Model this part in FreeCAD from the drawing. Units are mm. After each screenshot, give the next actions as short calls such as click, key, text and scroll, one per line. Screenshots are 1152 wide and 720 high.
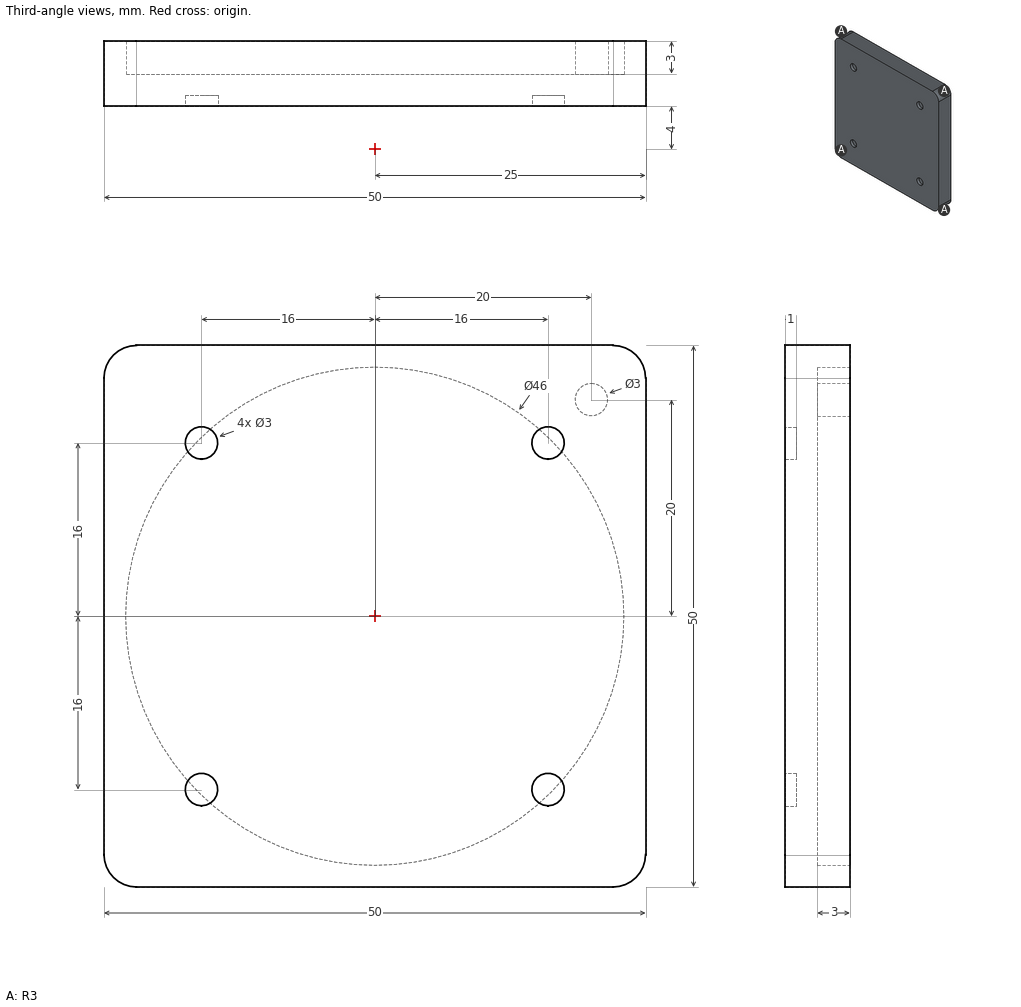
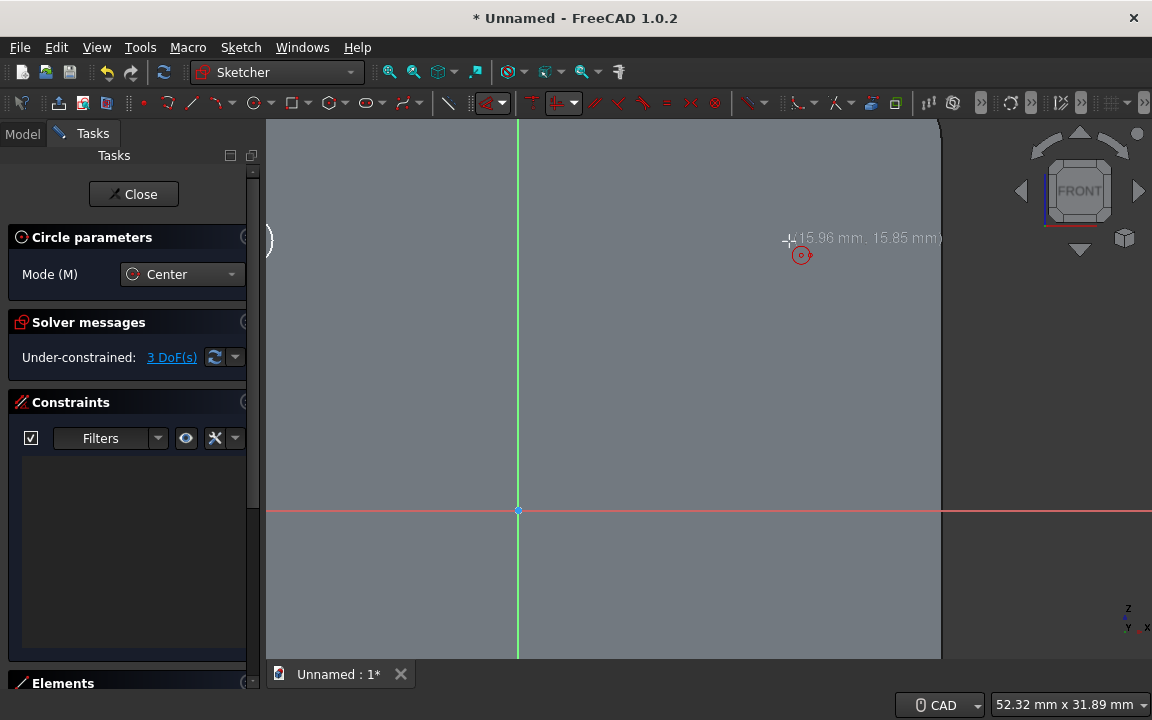
click(789, 240)
click(807, 222)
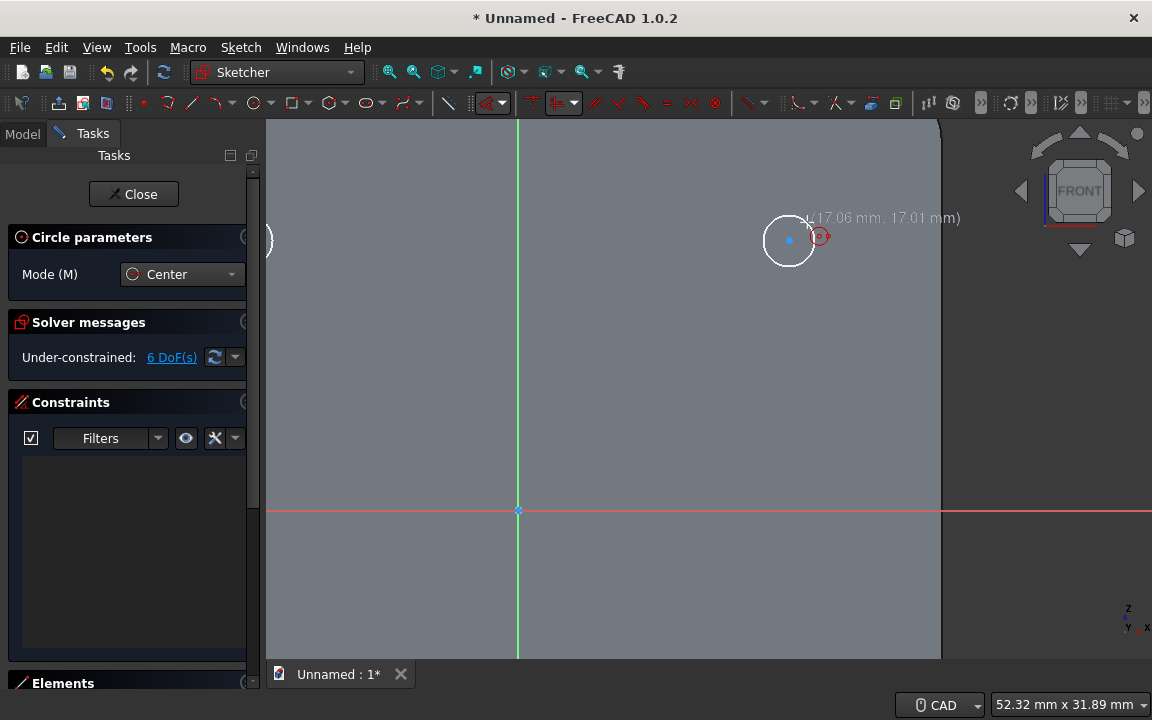
scroll(789, 241, down, 3)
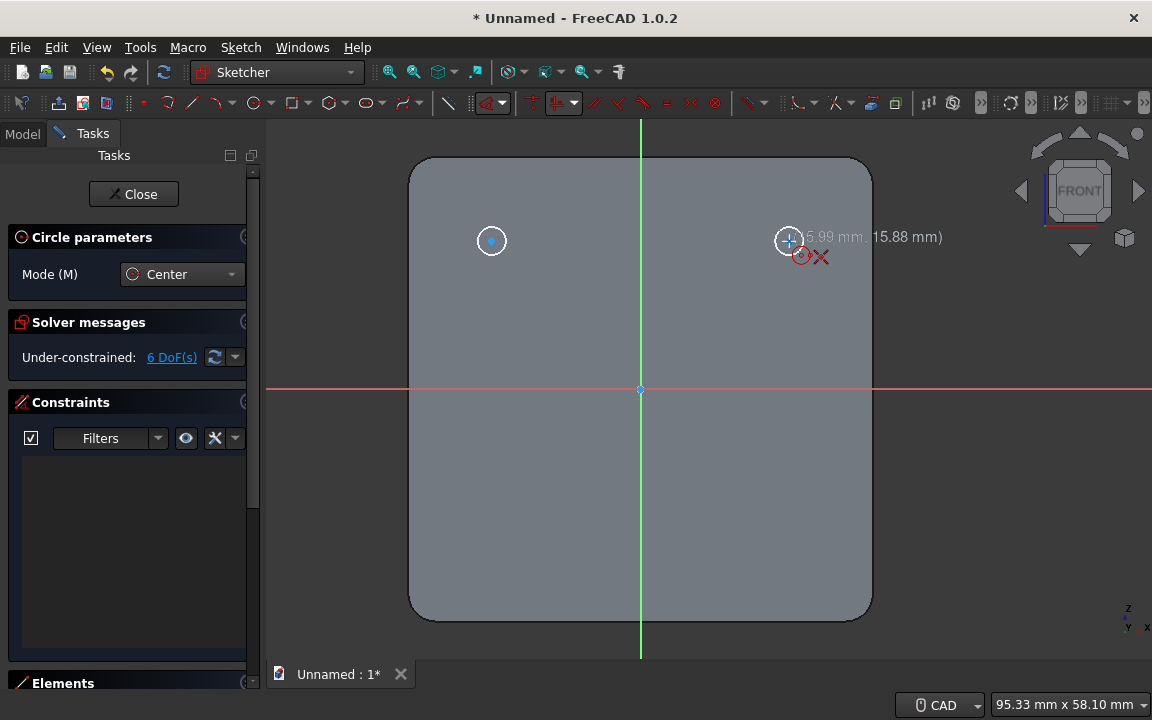
scroll(492, 538, up, 3)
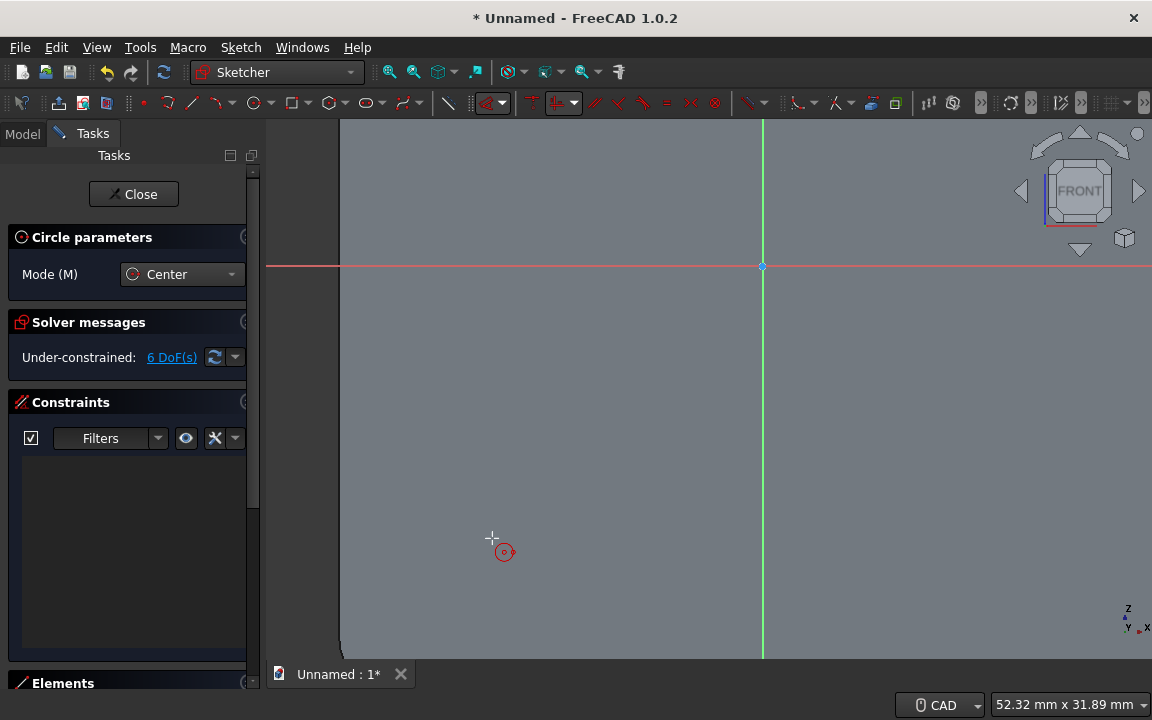
click(492, 537)
click(510, 519)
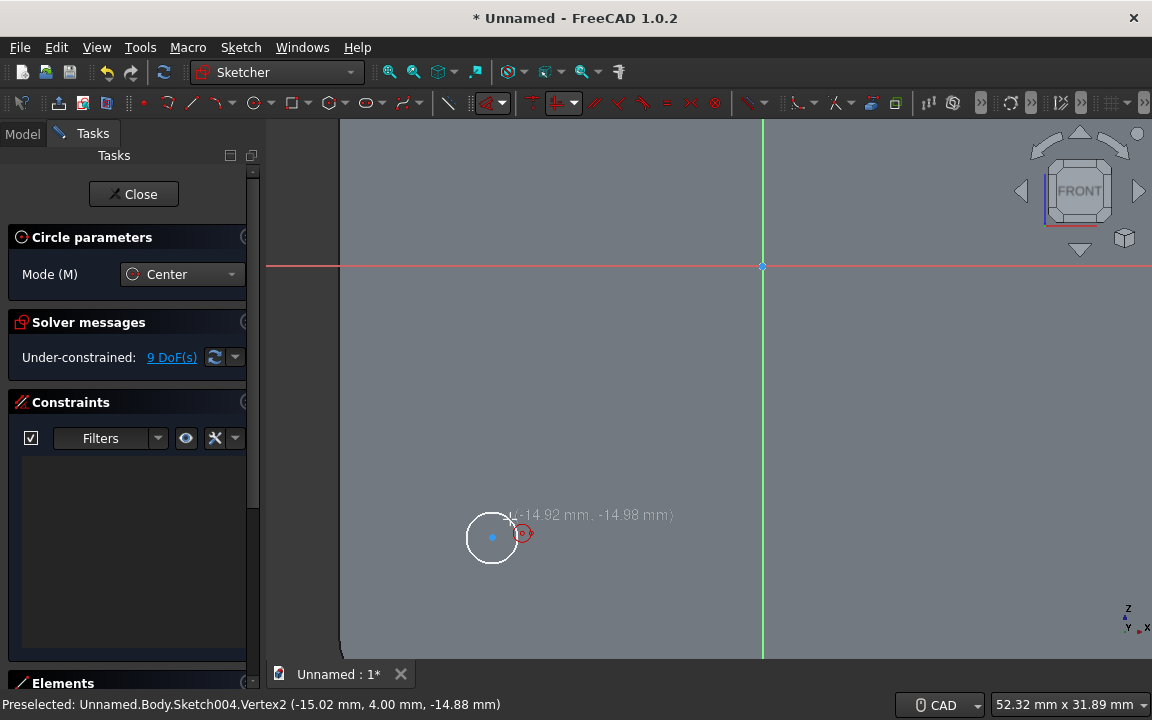
scroll(492, 538, down, 3)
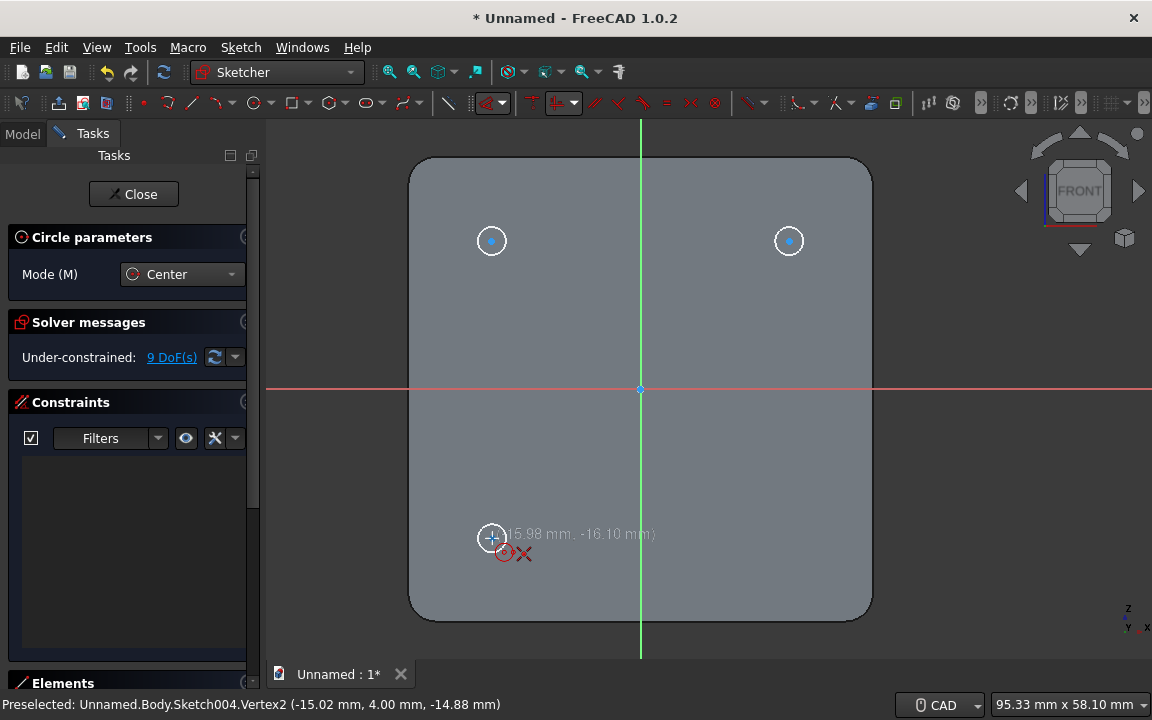
scroll(789, 538, up, 3)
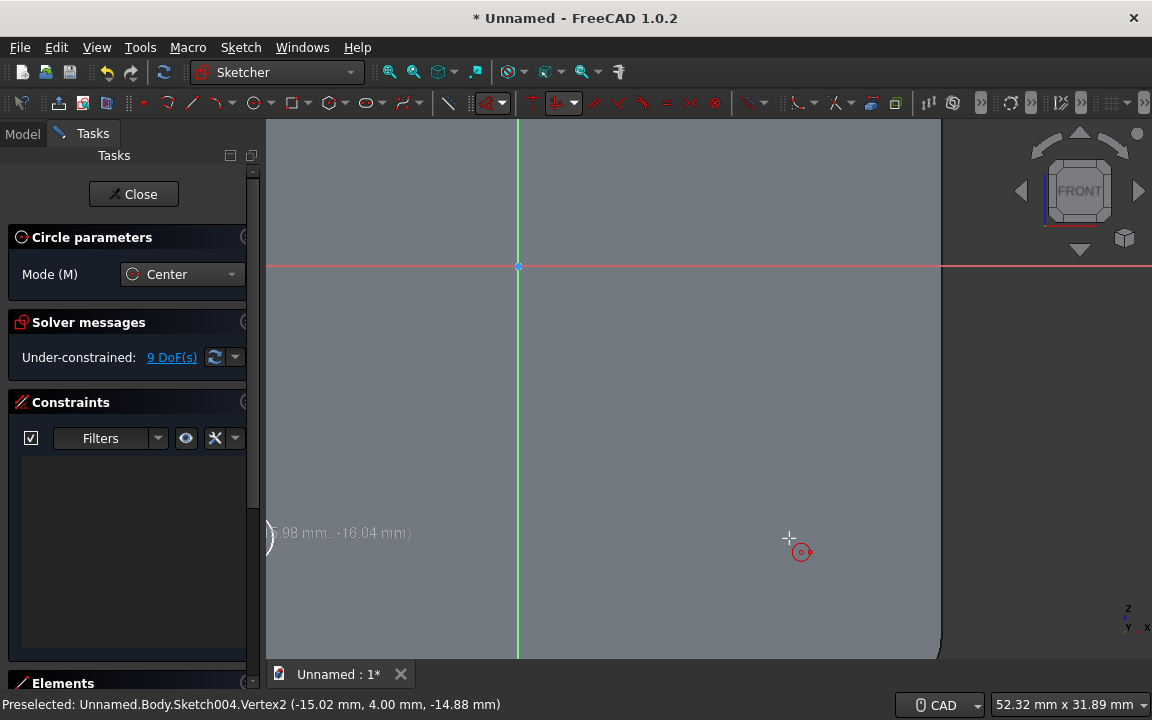
click(789, 537)
click(807, 519)
key(Escape)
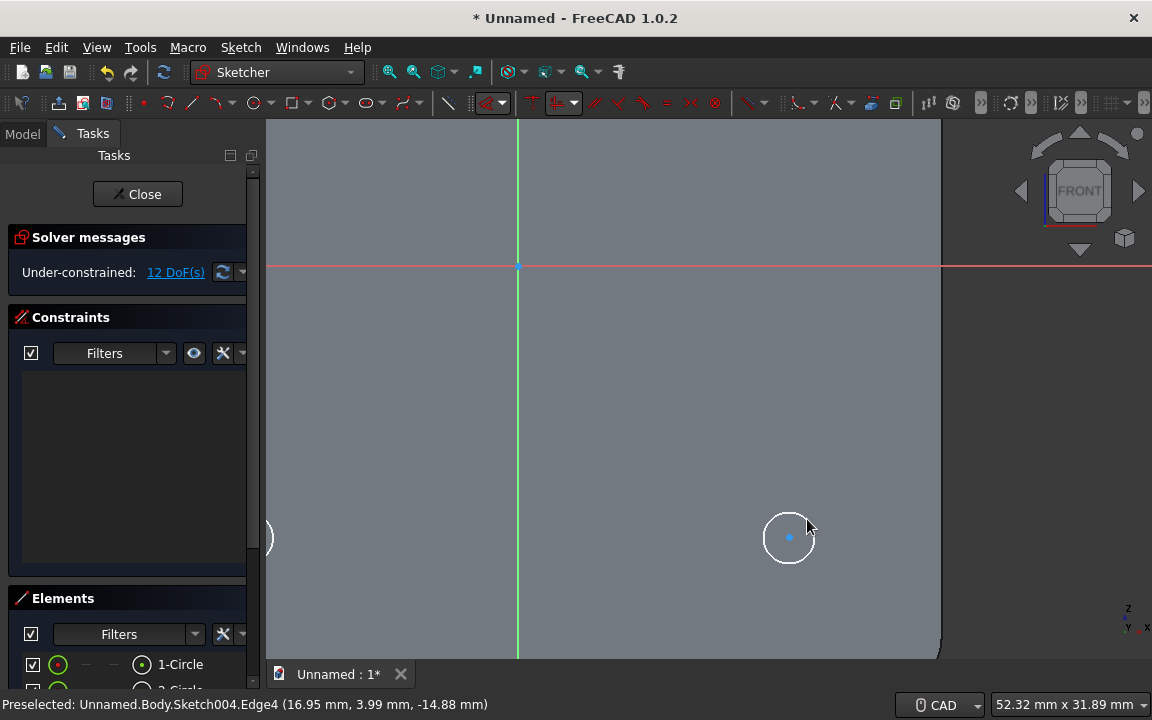
scroll(789, 538, down, 3)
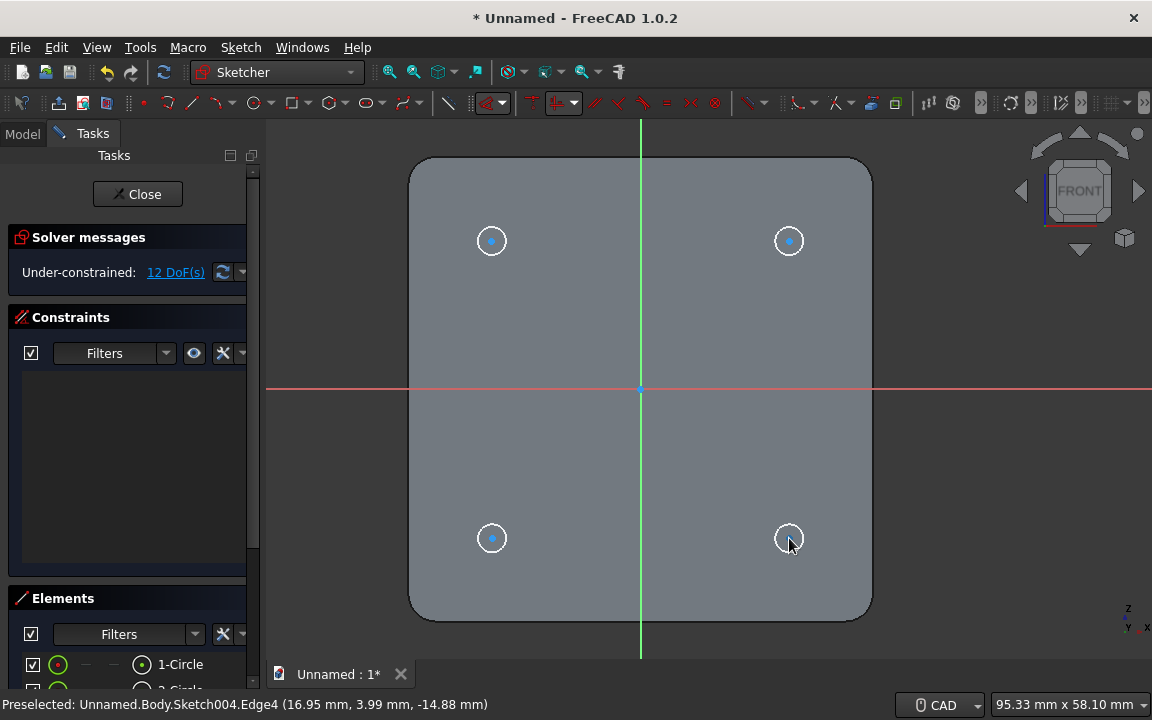
click(502, 231)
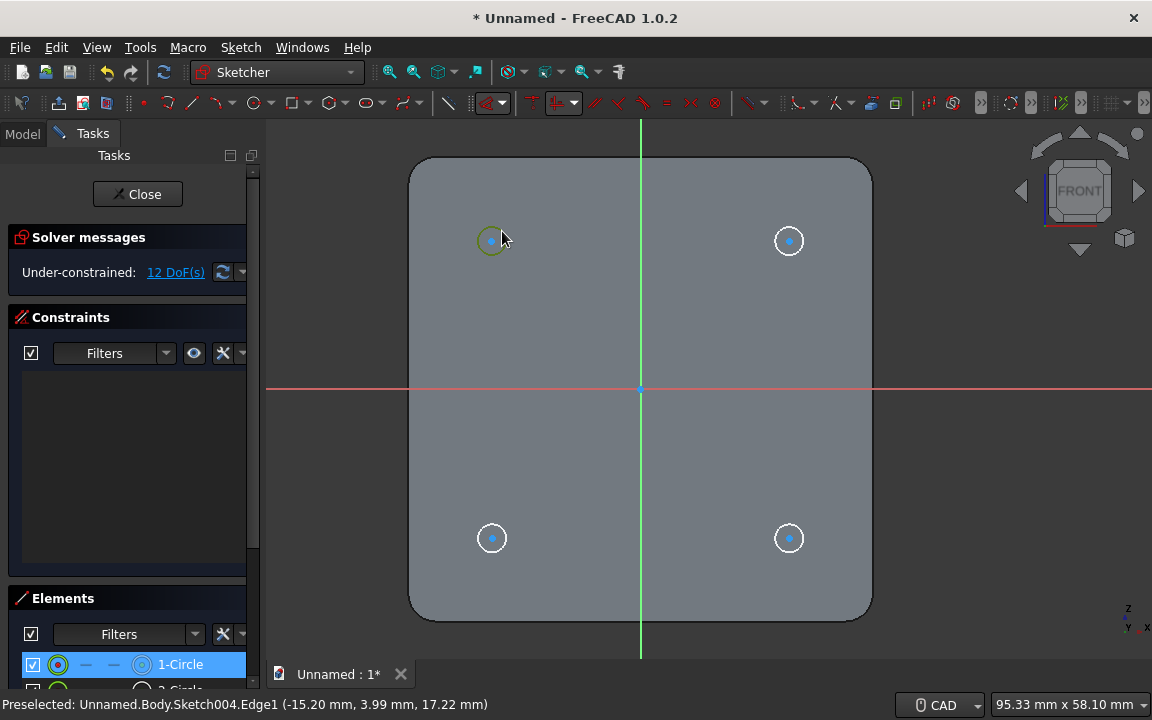
click(799, 231)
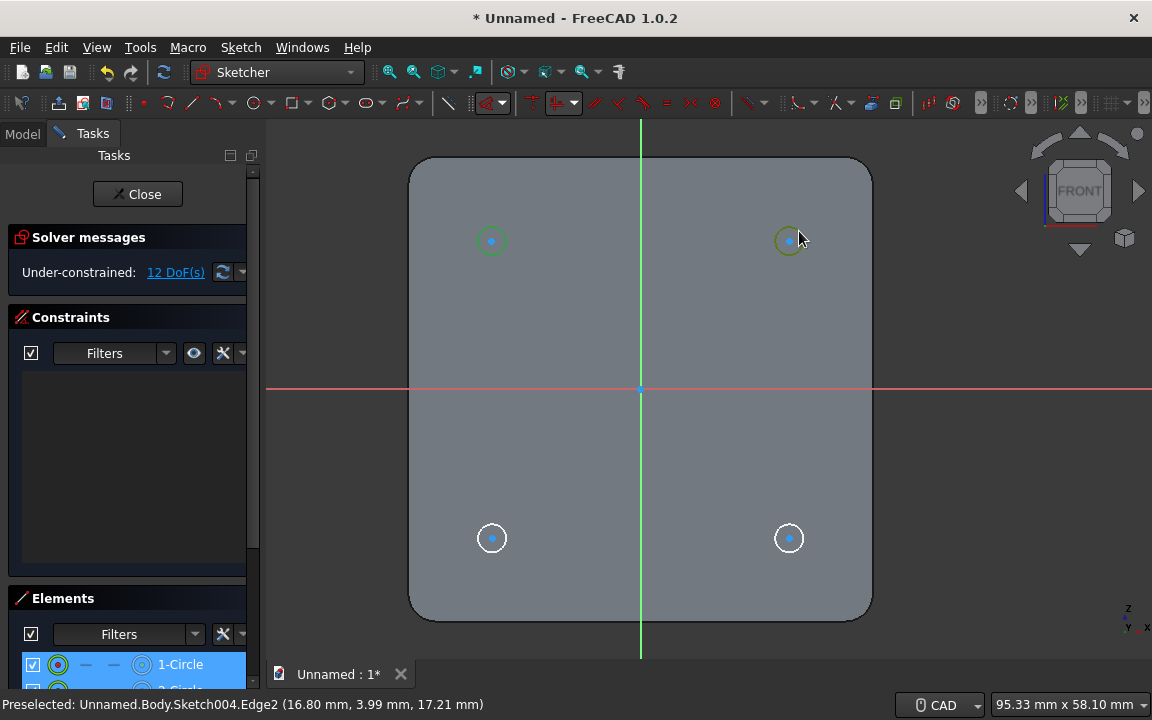
click(502, 528)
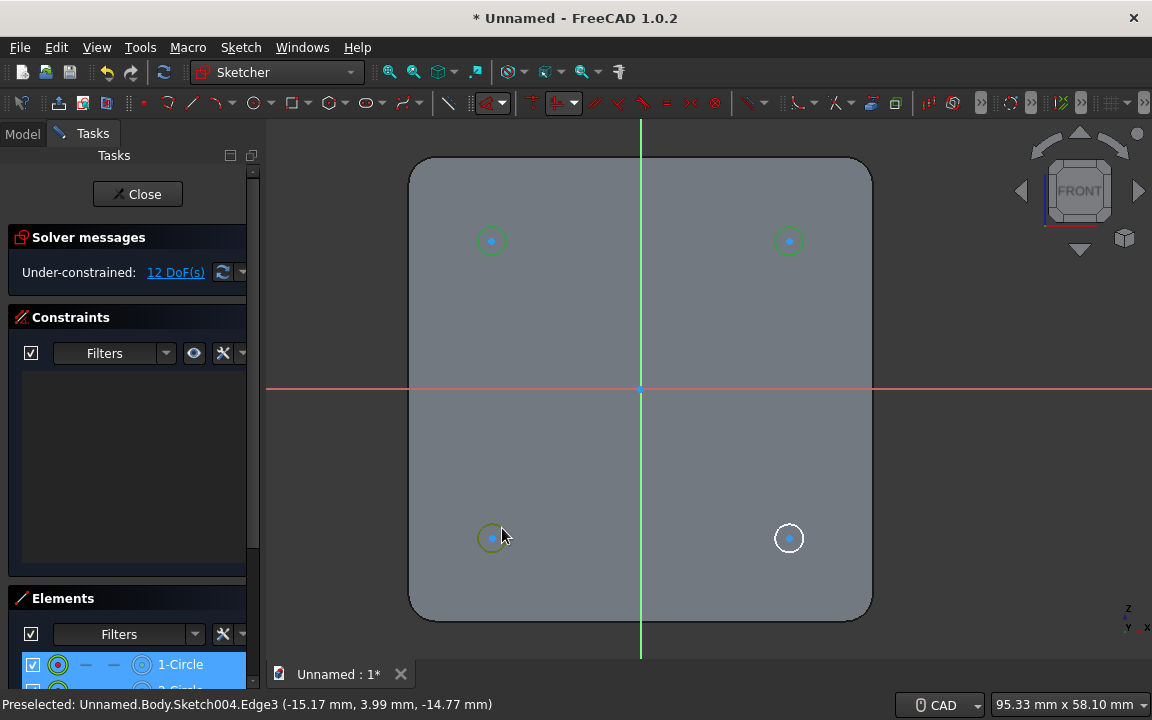
click(799, 528)